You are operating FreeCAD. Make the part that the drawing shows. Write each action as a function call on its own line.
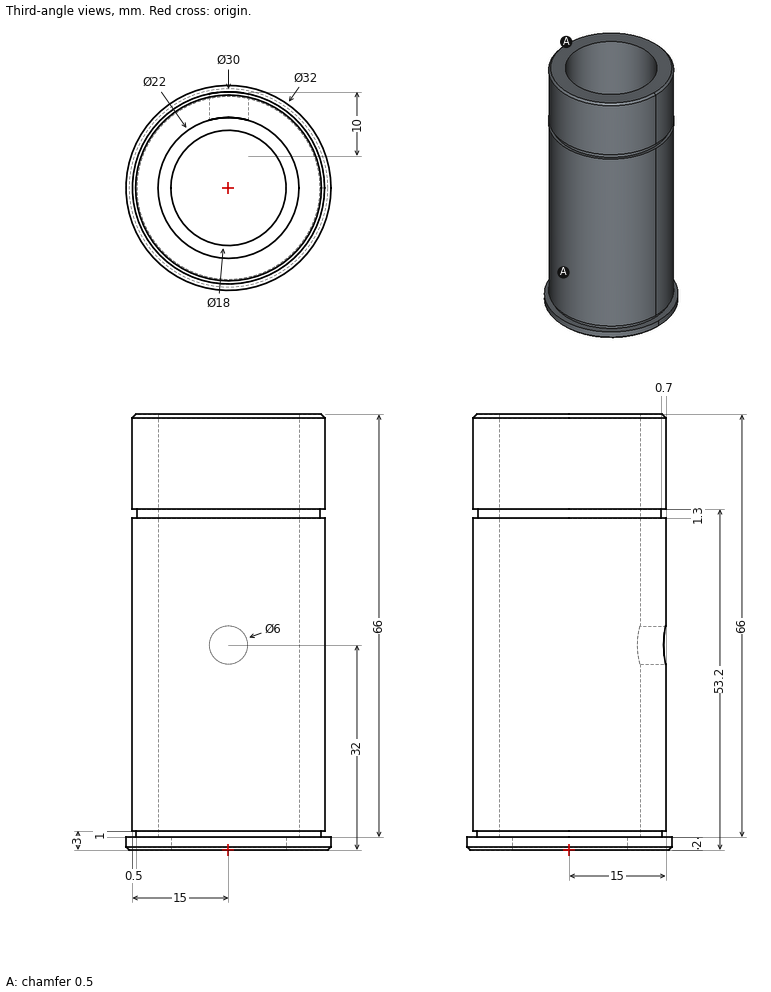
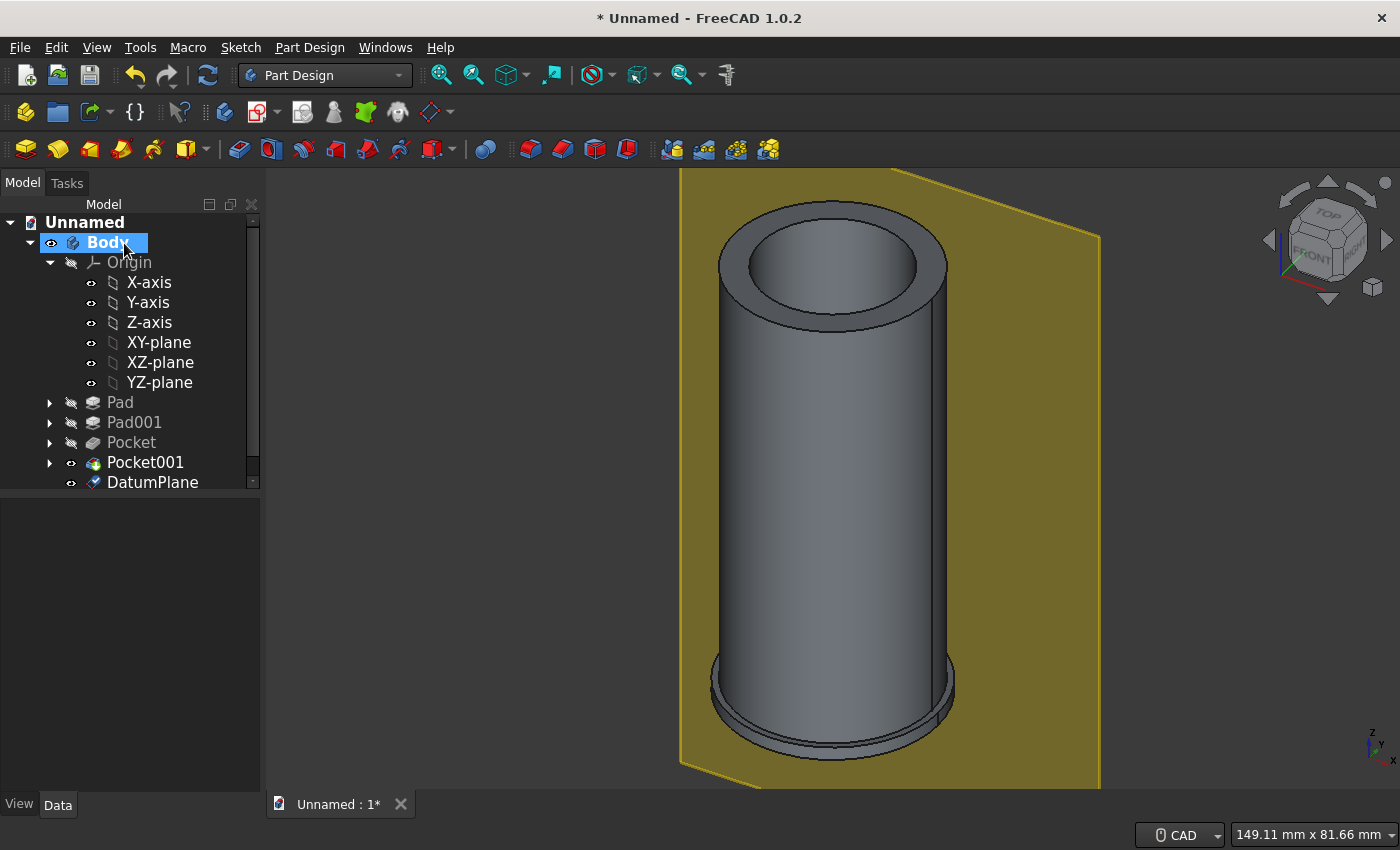
click(116, 483)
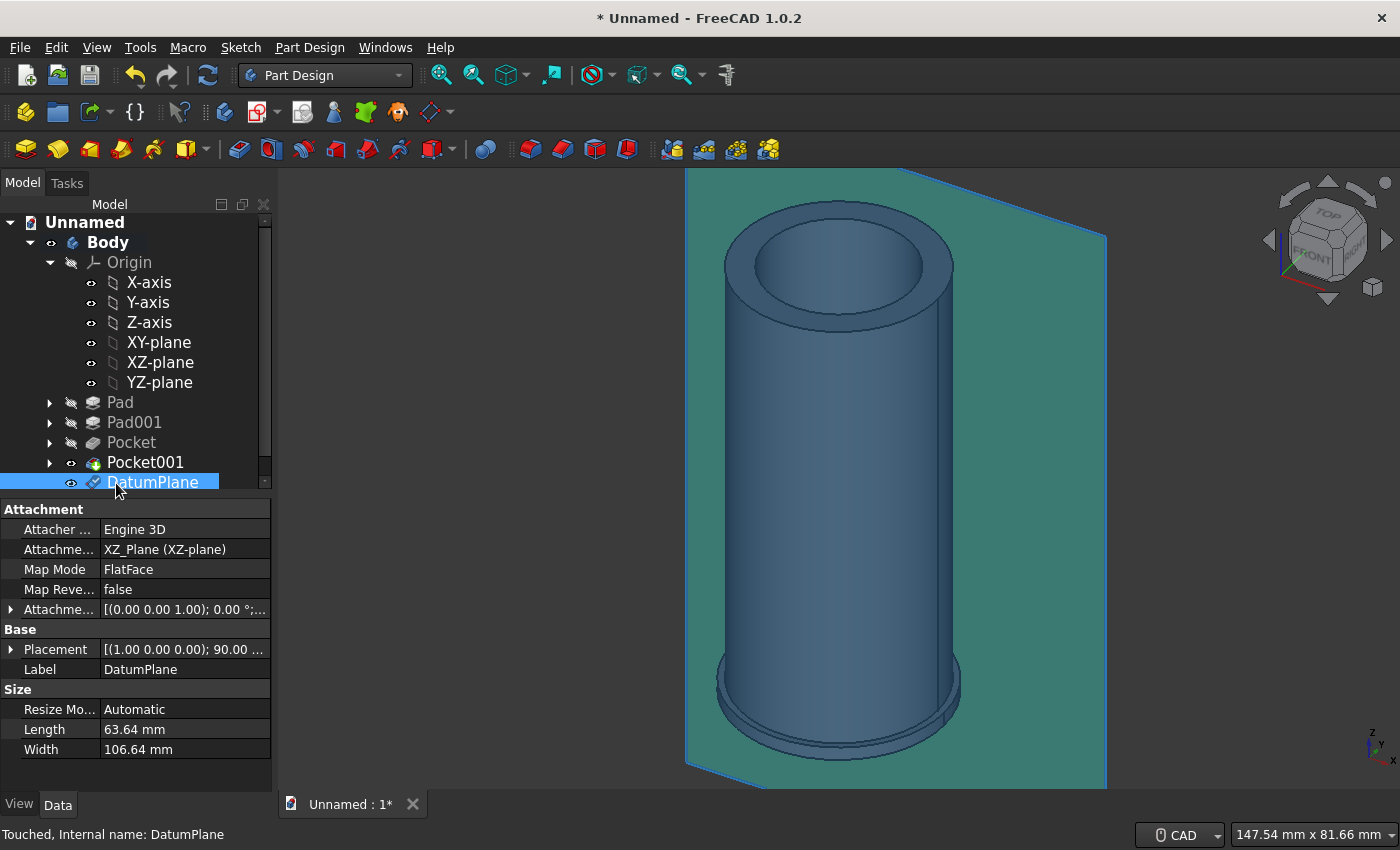
click(258, 112)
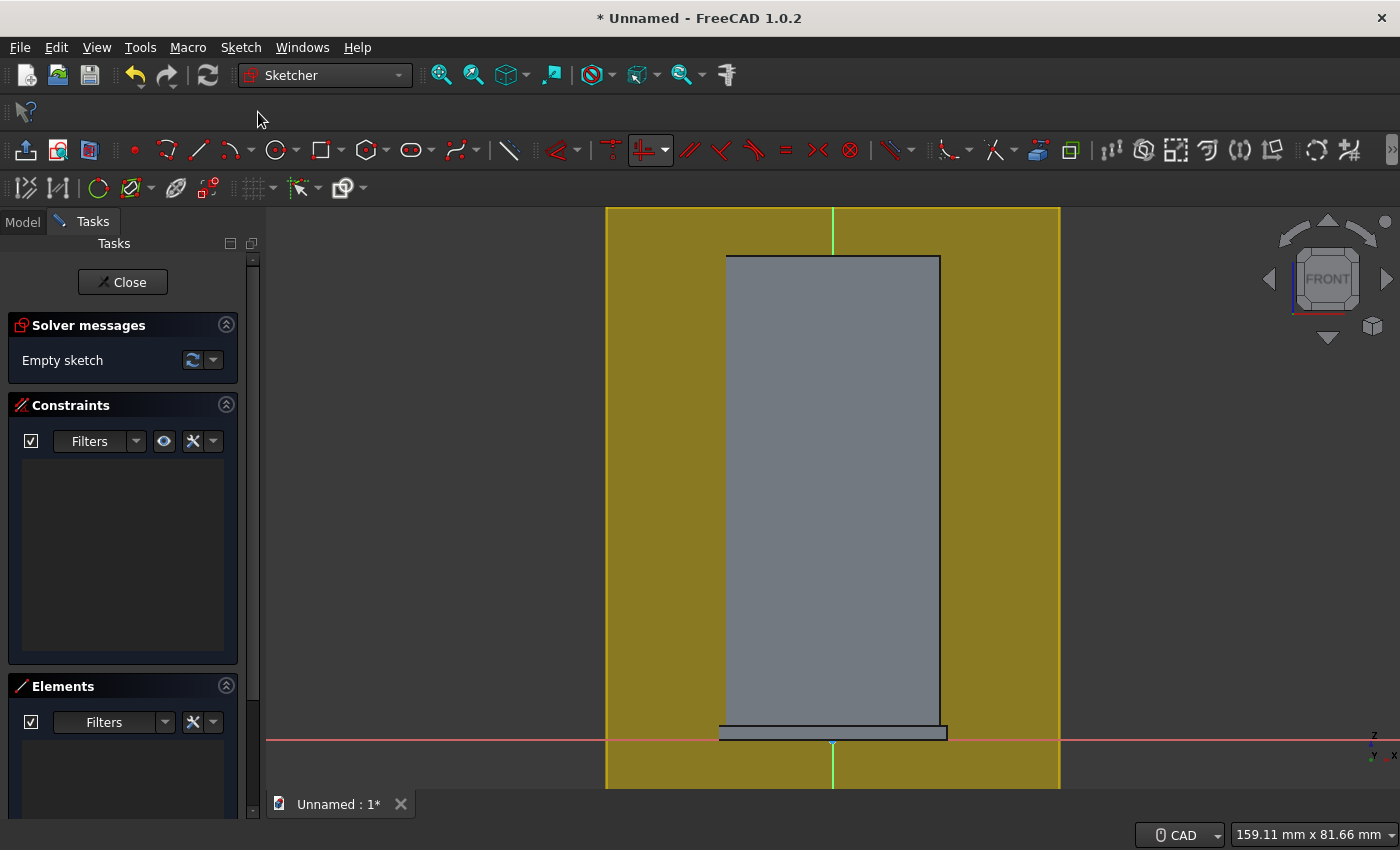
click(90, 150)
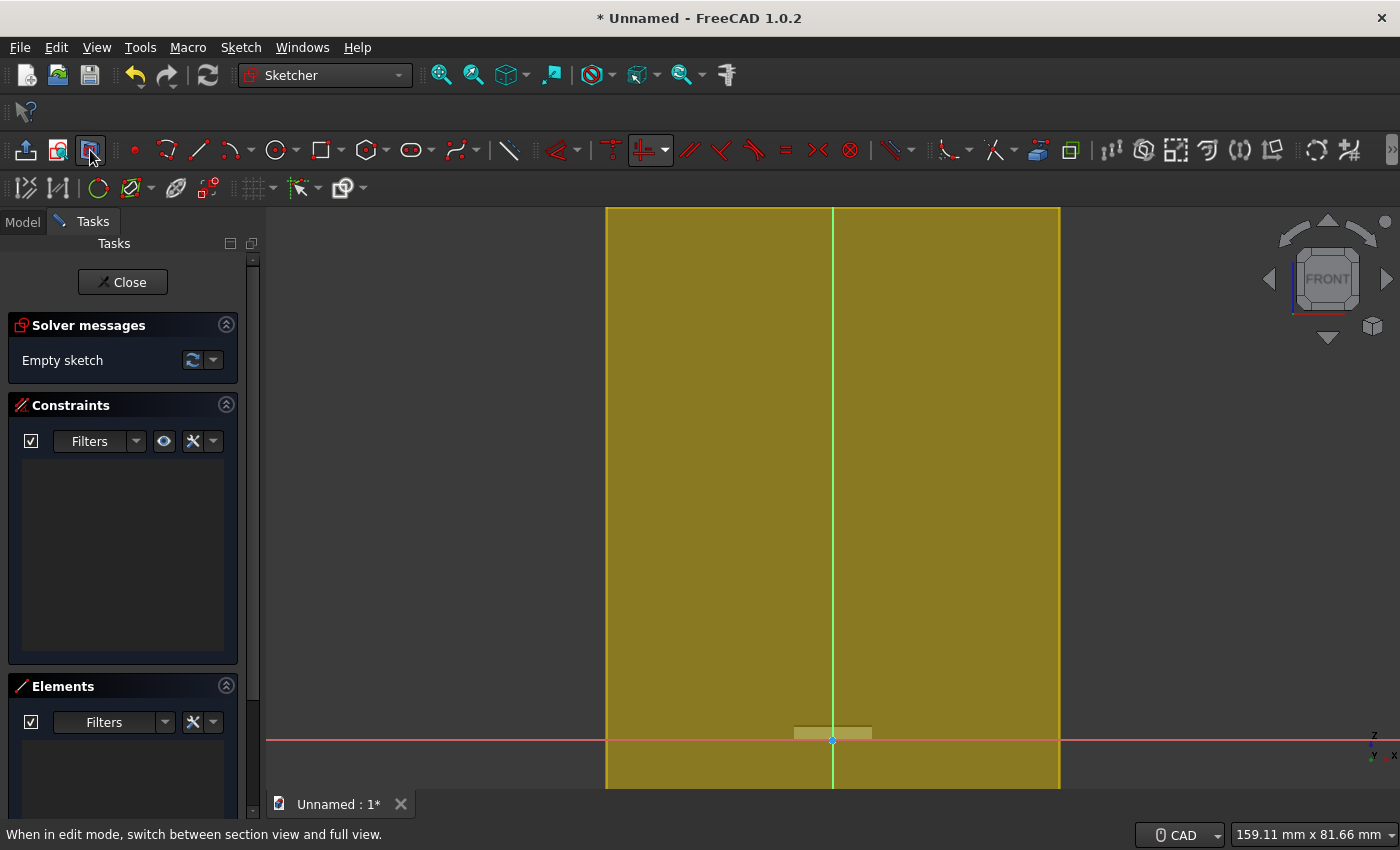
scroll(841, 514, up, 11)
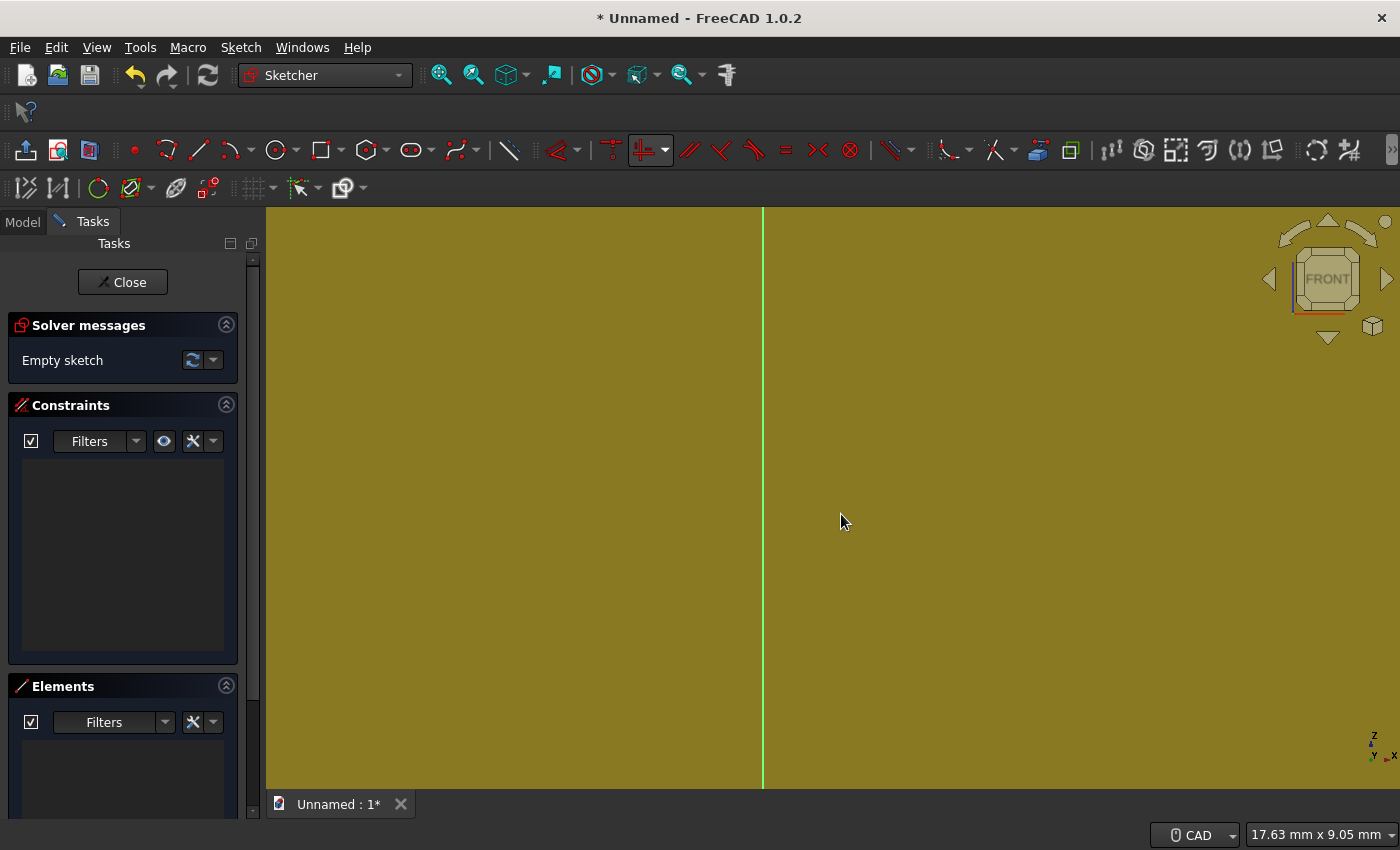
click(276, 150)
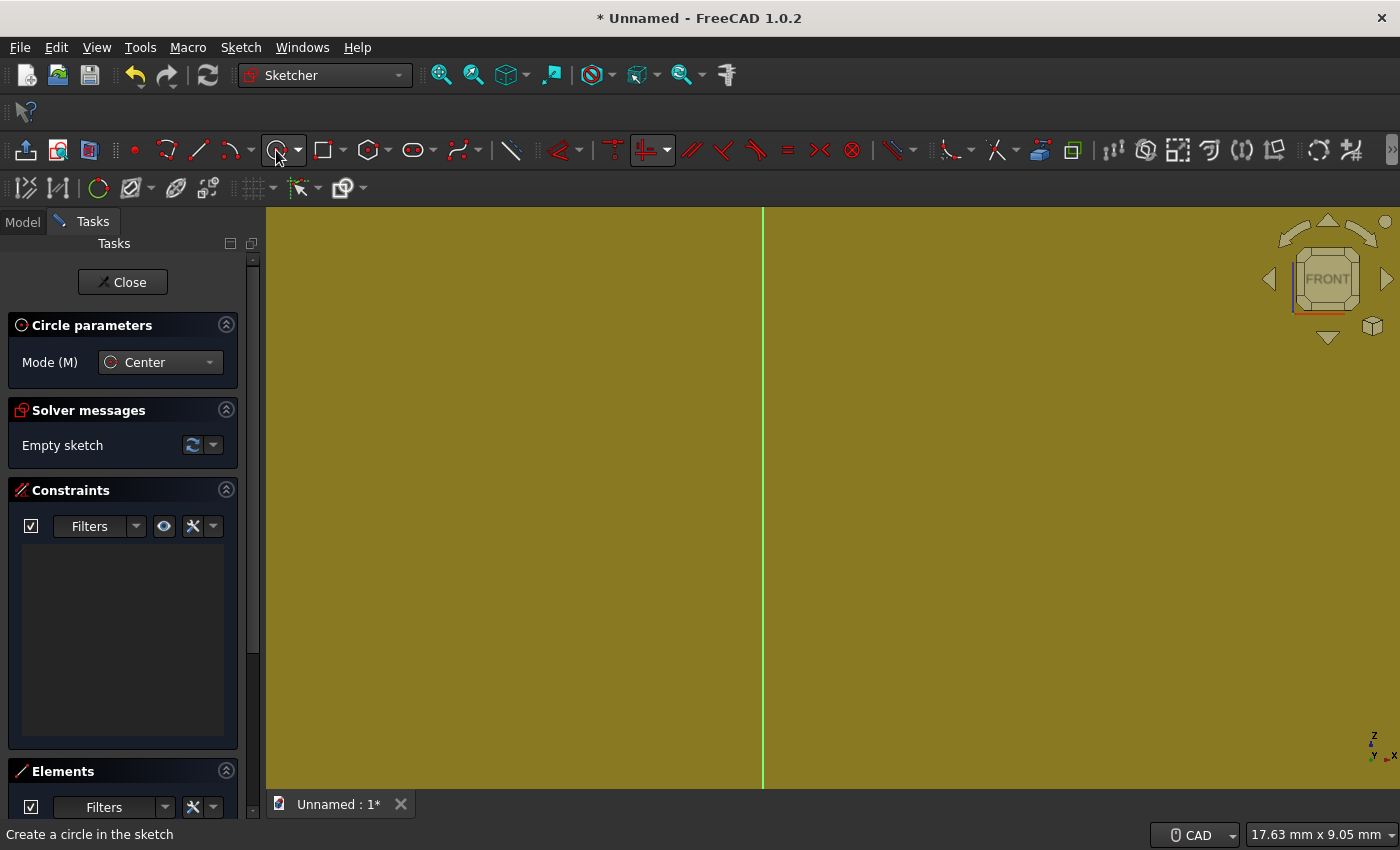
click(763, 494)
move(900, 358)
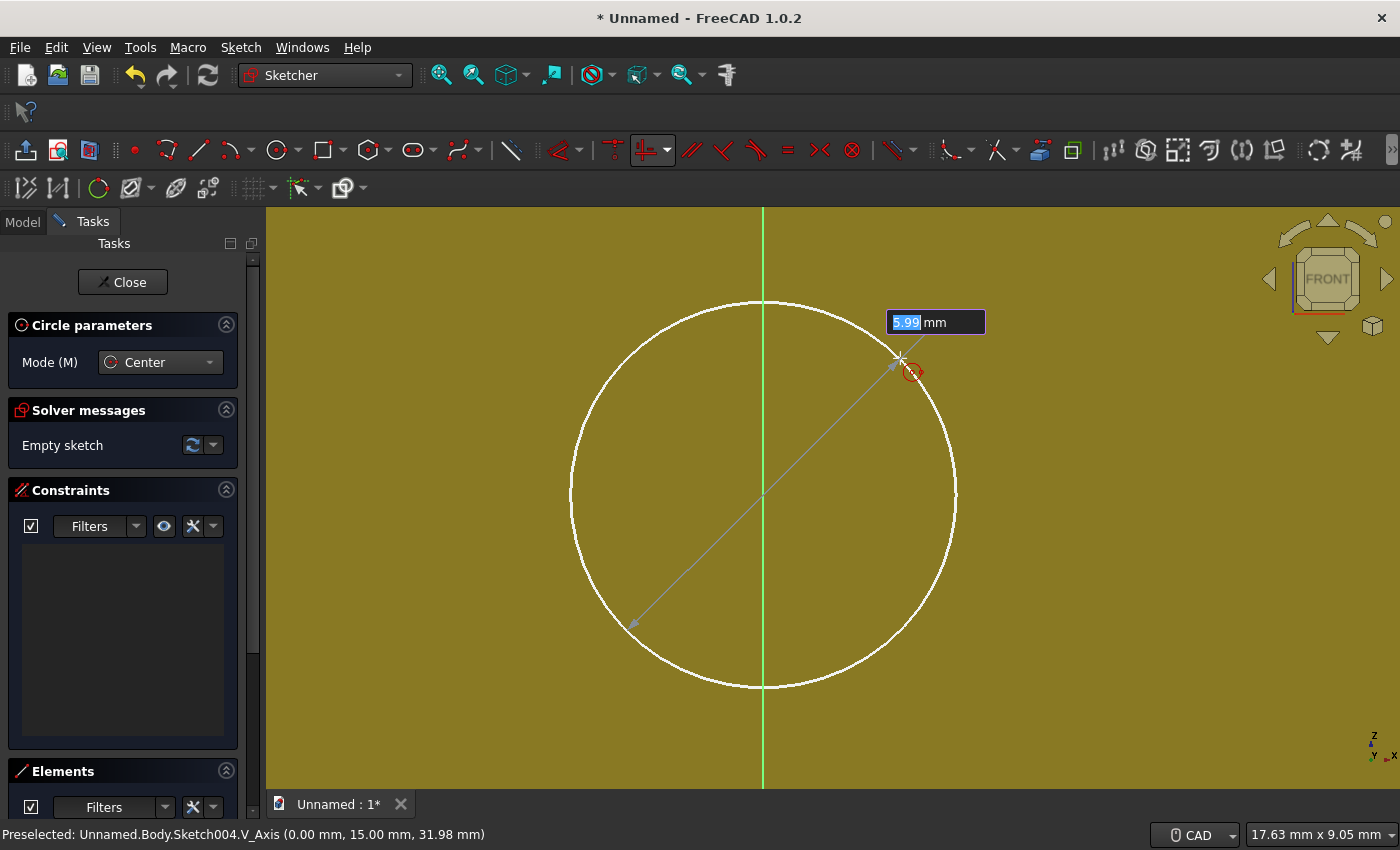
text(6)
key(Return)
key(Escape)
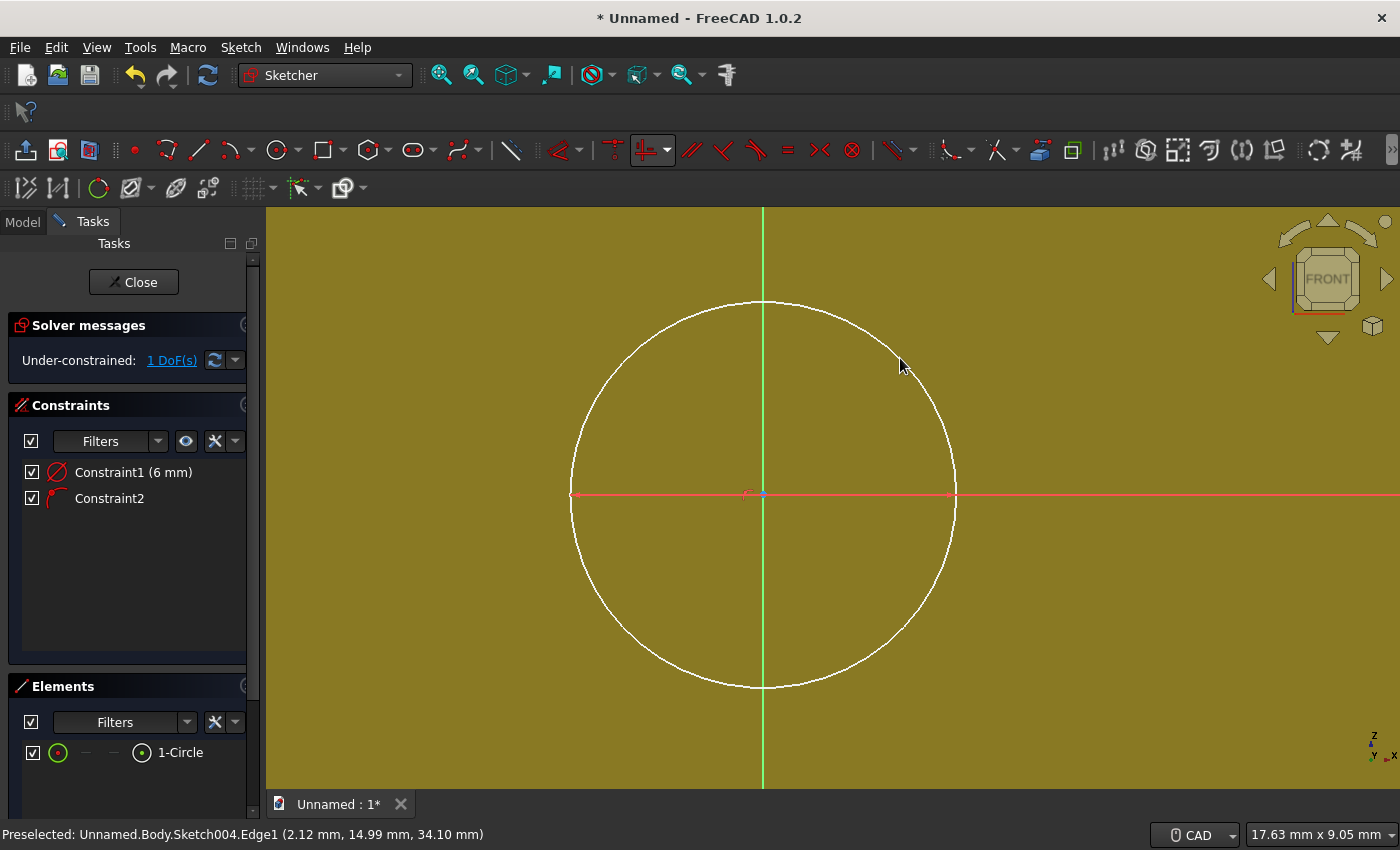
key(d)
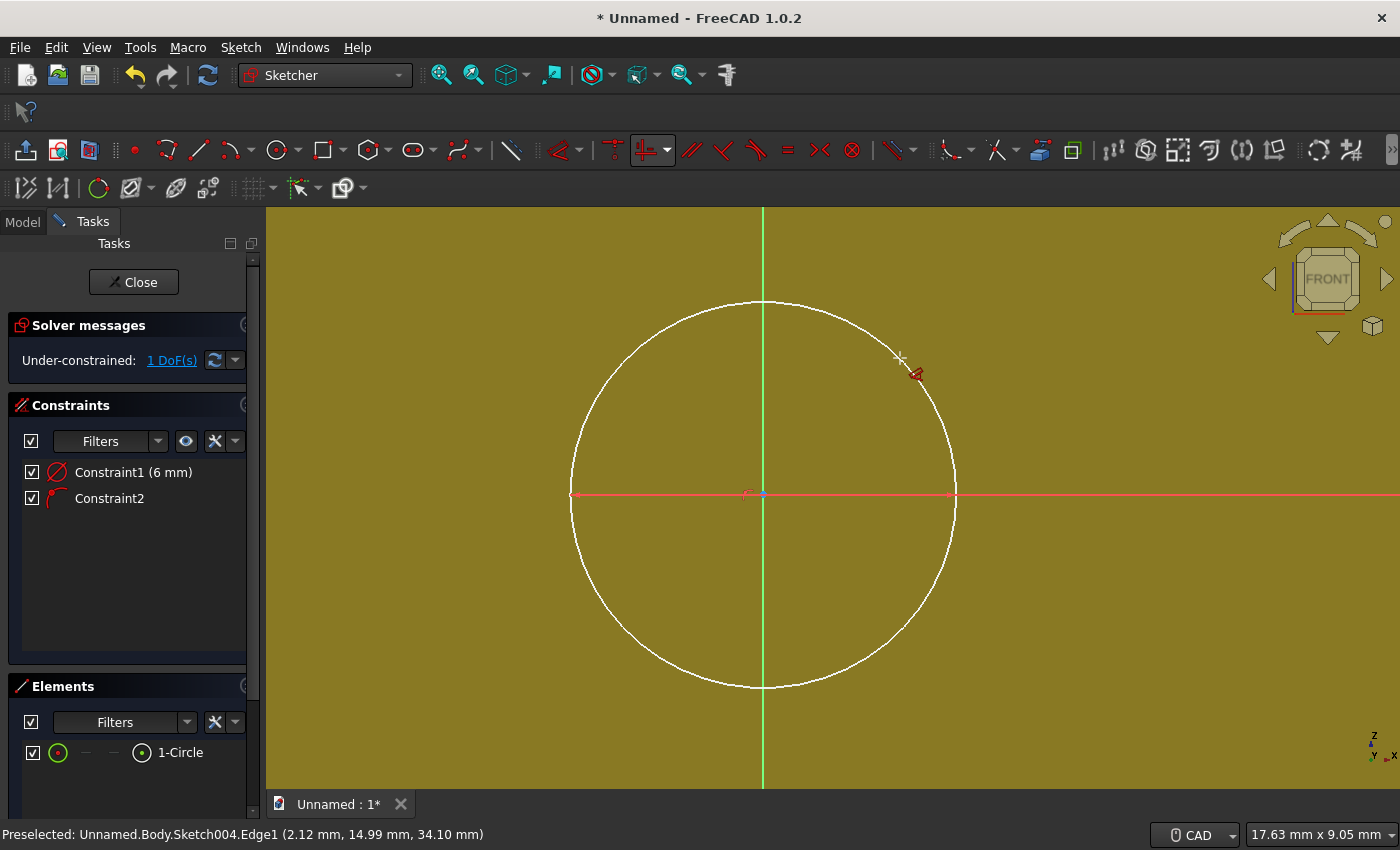
click(763, 495)
click(797, 628)